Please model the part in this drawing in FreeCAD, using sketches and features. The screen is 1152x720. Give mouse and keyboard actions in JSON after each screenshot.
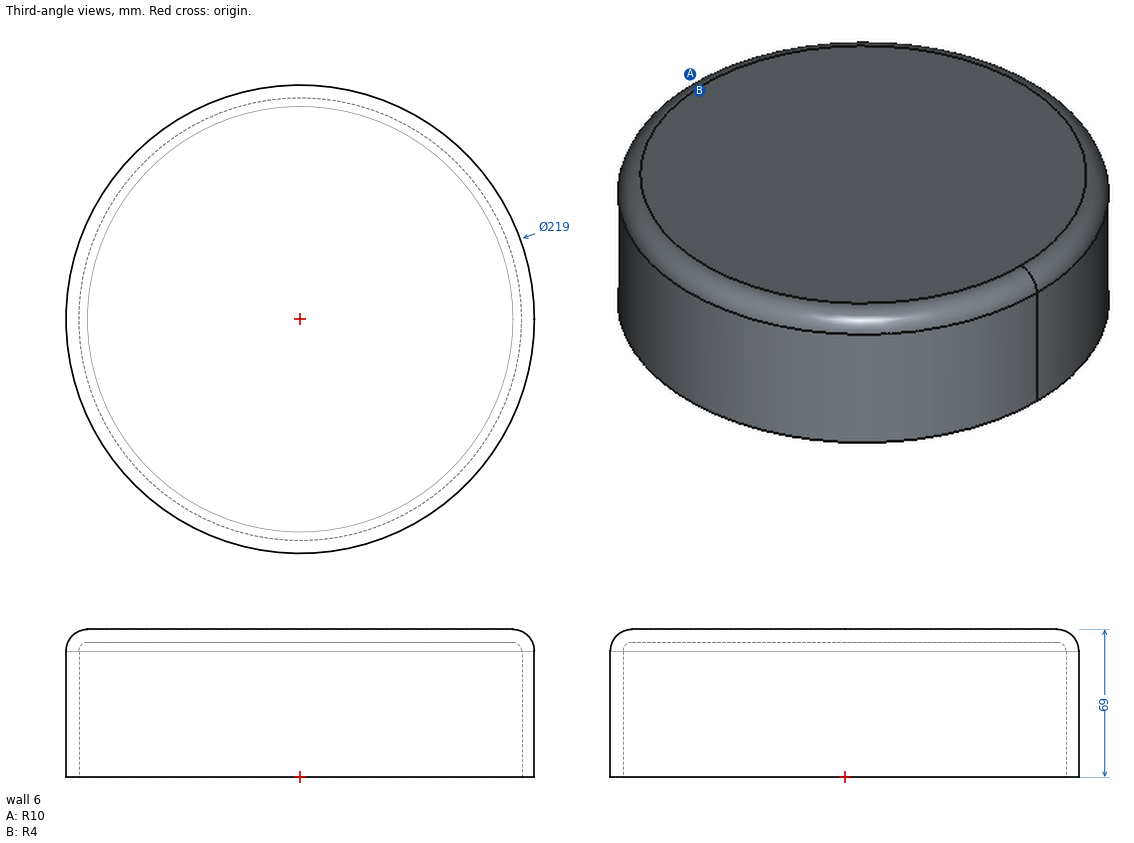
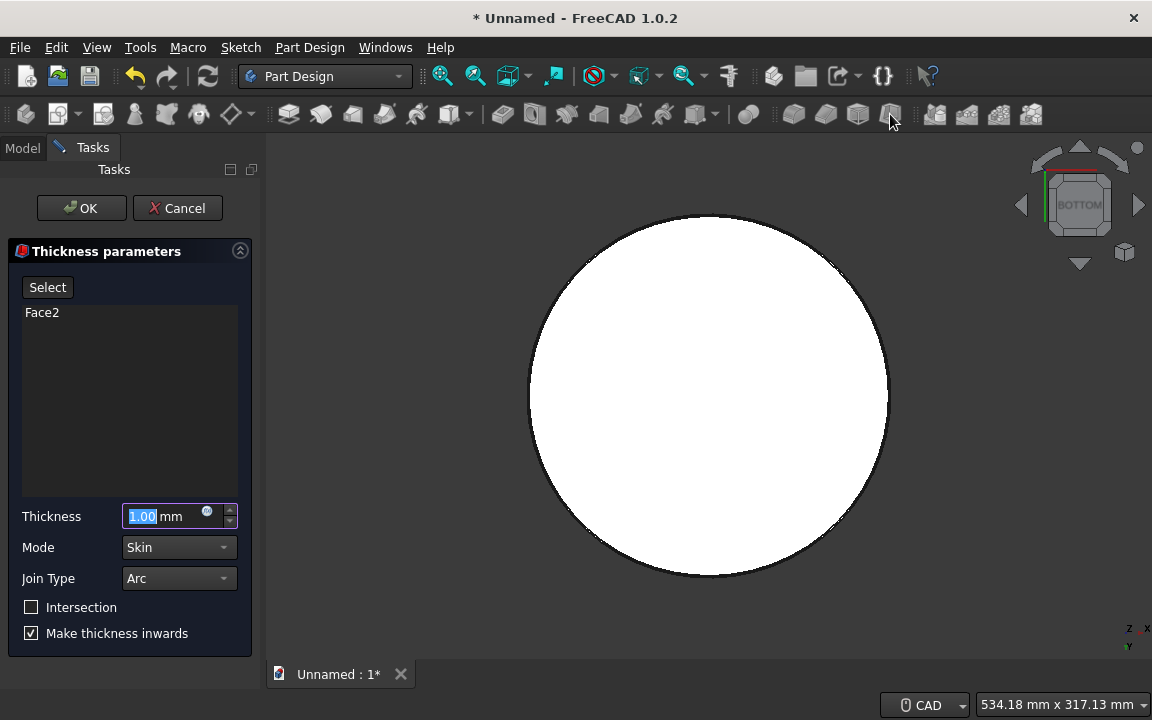
{"action": "type", "text": "6"}
{"action": "key", "text": "Tab"}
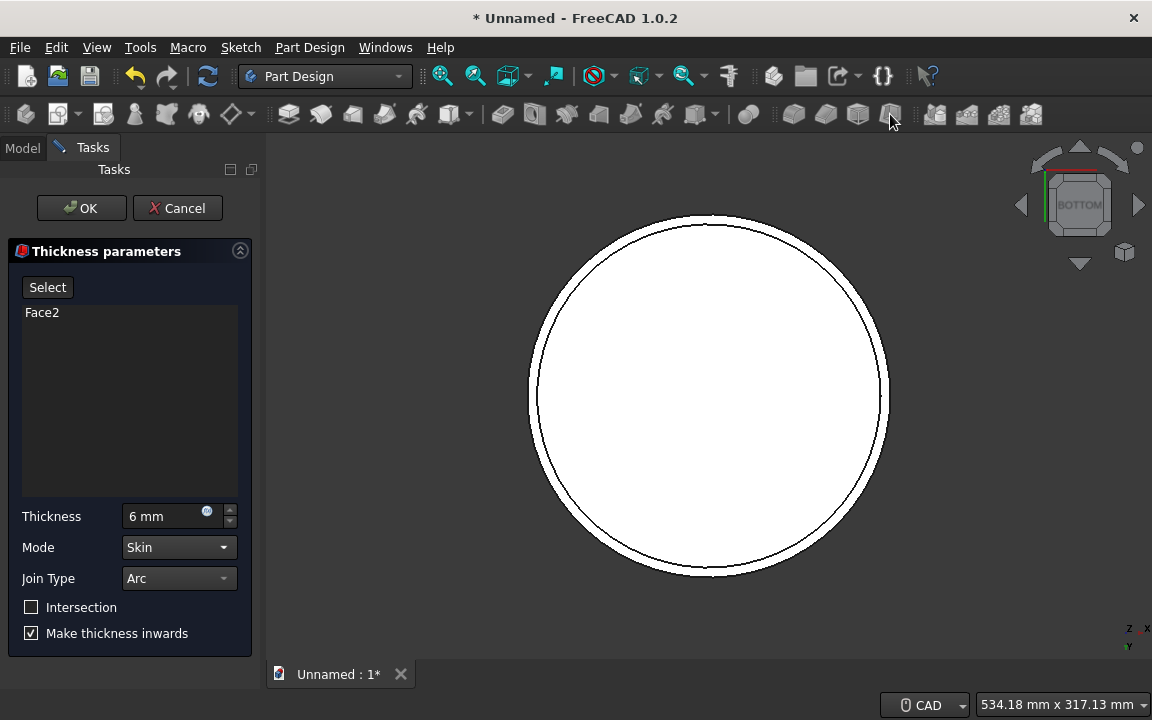
{"action": "left_click", "coordinate": [180, 578]}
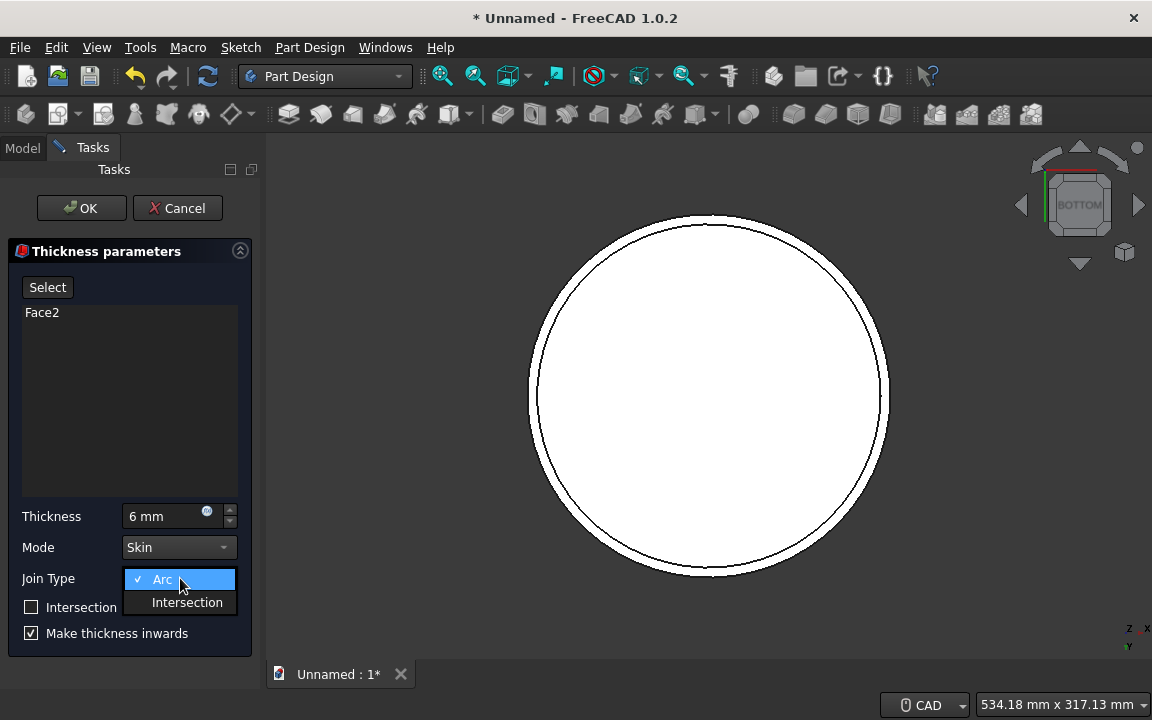
{"action": "left_click", "coordinate": [179, 602]}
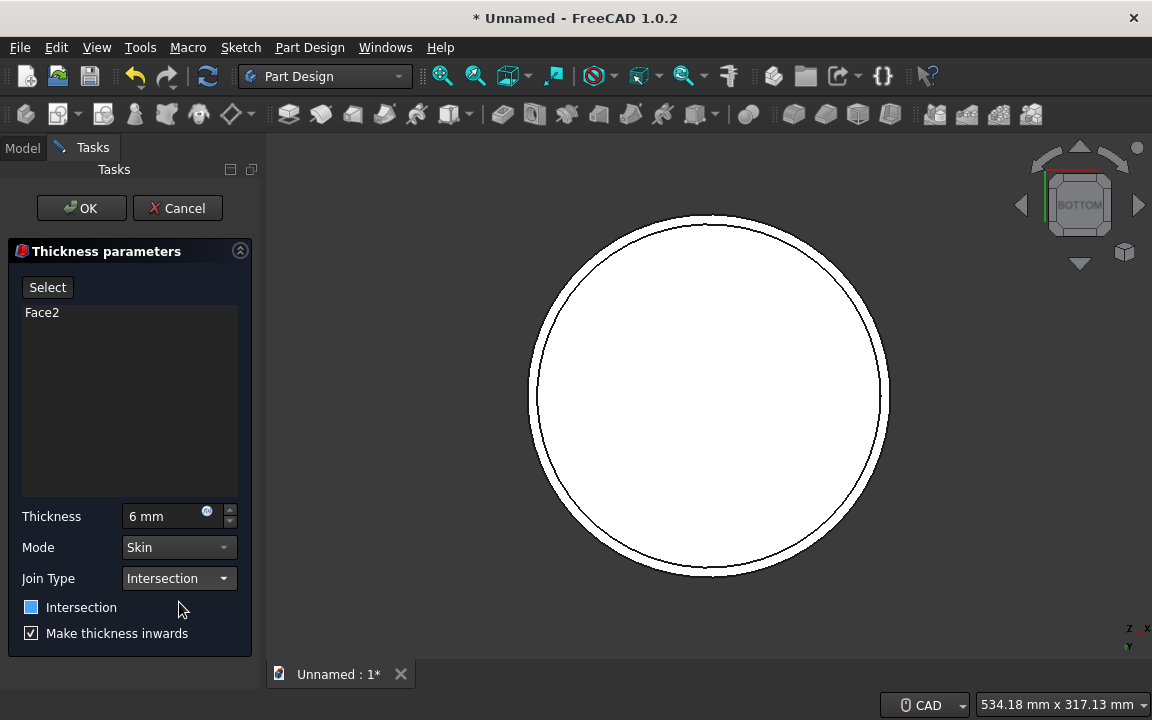
{"action": "left_click", "coordinate": [82, 208]}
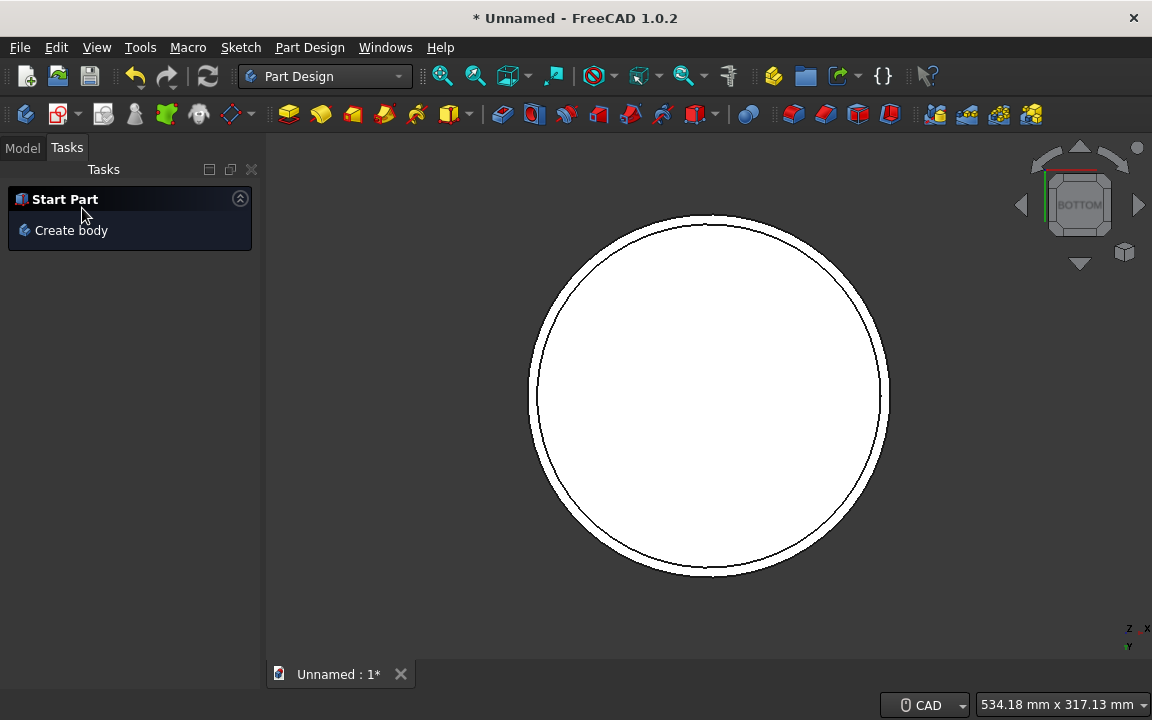
{"action": "key", "text": "0"}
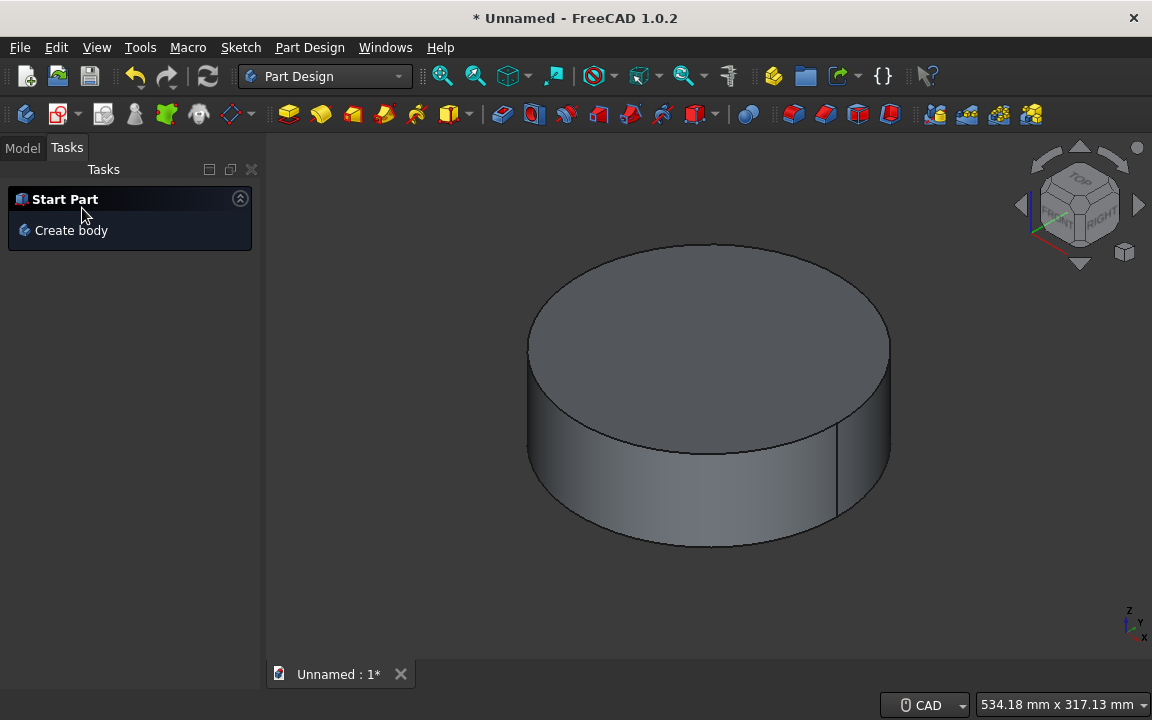
{"action": "left_click", "coordinate": [547, 396]}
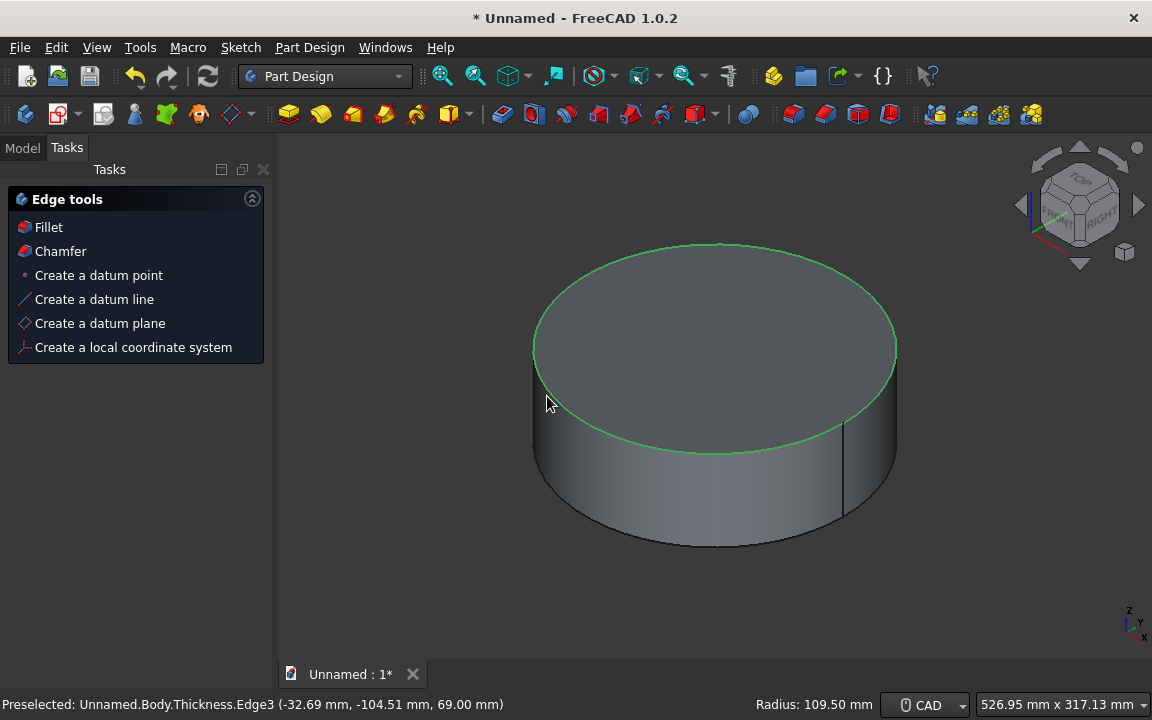
{"action": "left_click", "coordinate": [794, 114]}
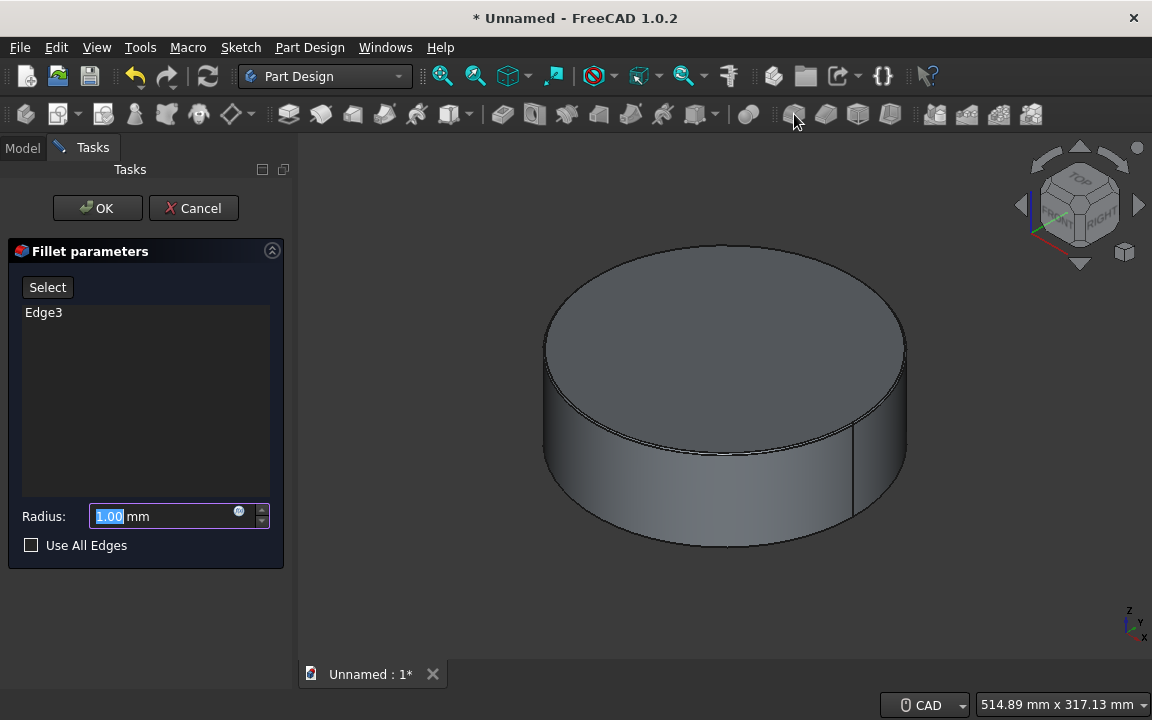
{"action": "type", "text": "10"}
{"action": "key", "text": "Tab"}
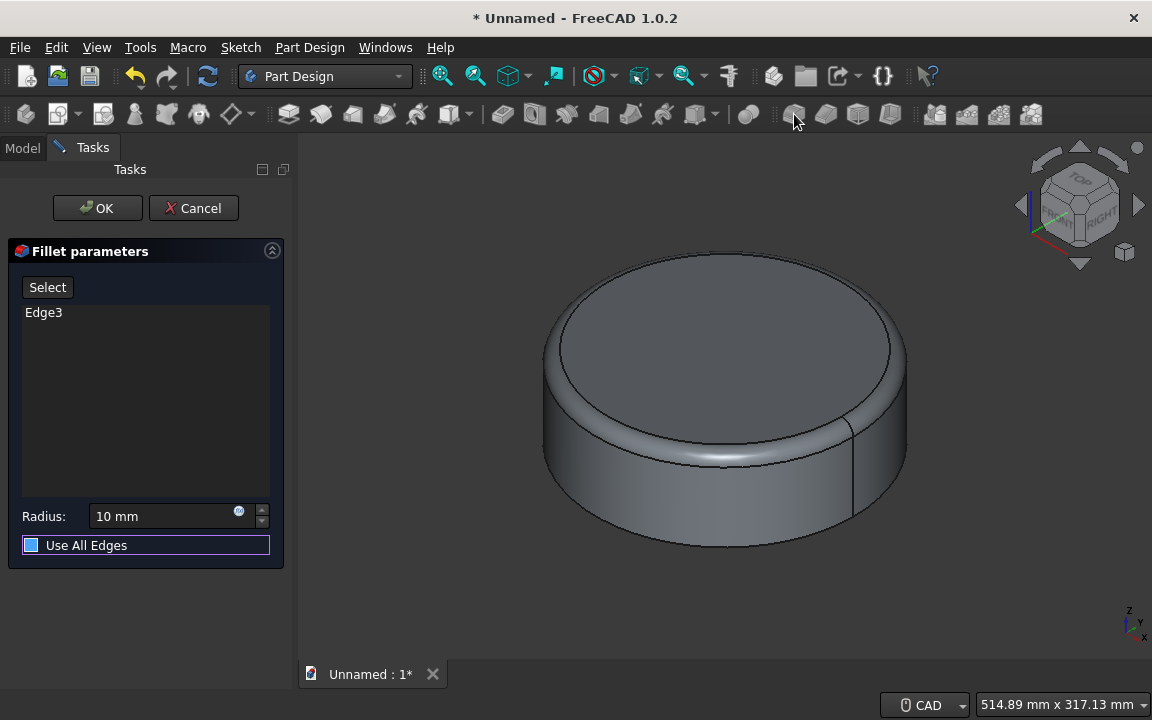
{"action": "left_click", "coordinate": [98, 208]}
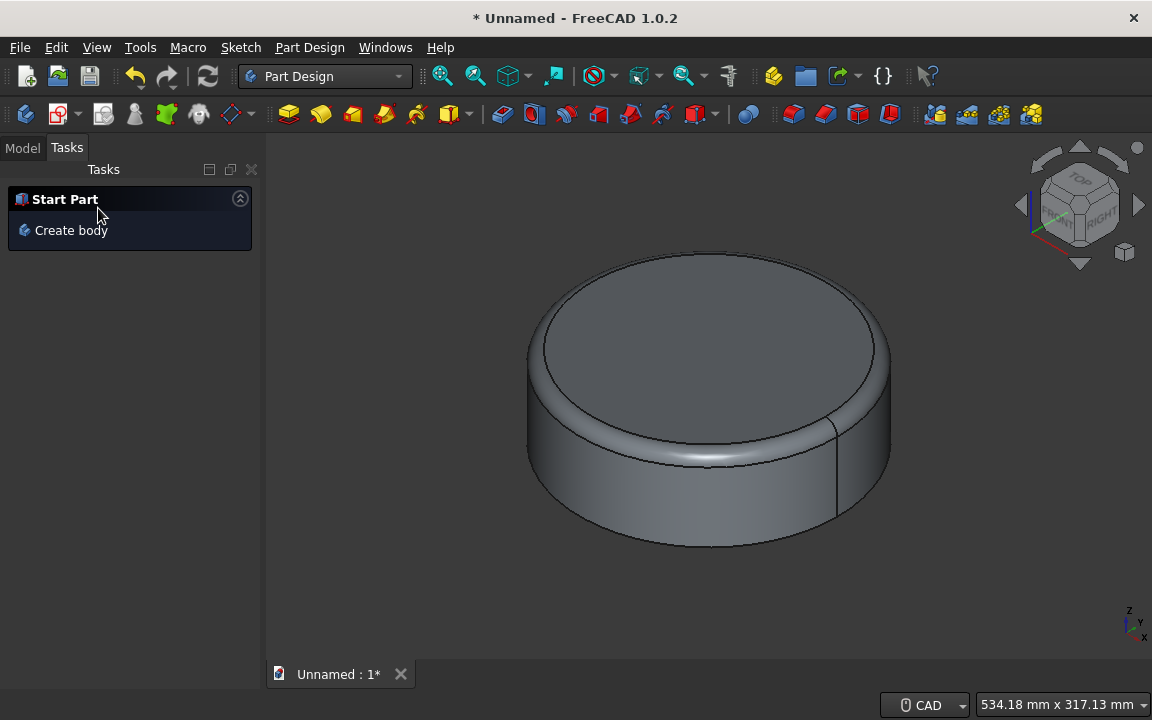
{"action": "key", "text": "2"}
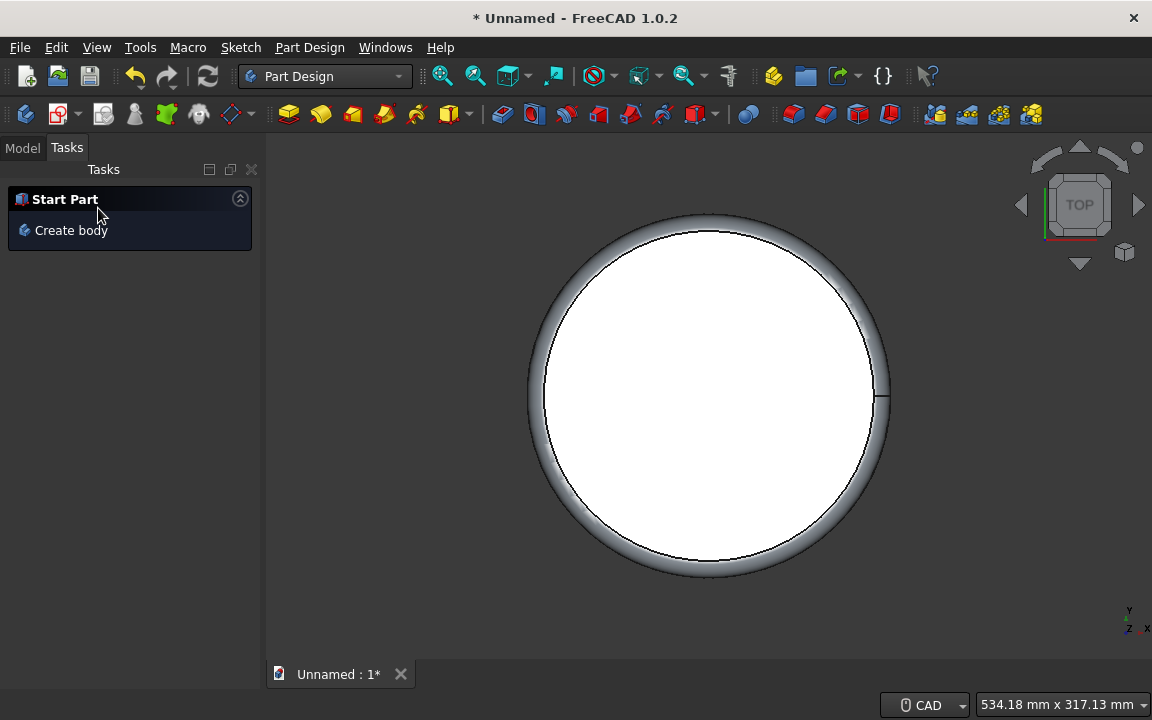
{"action": "key", "text": "0"}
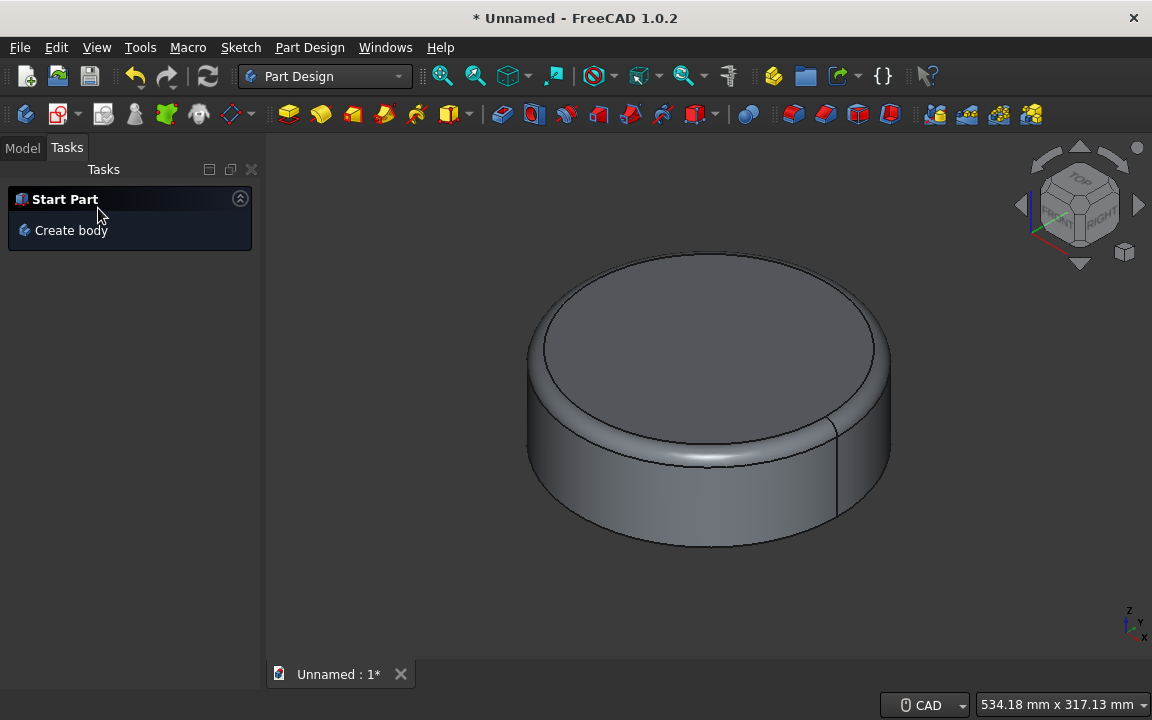
{"action": "key", "text": "1"}